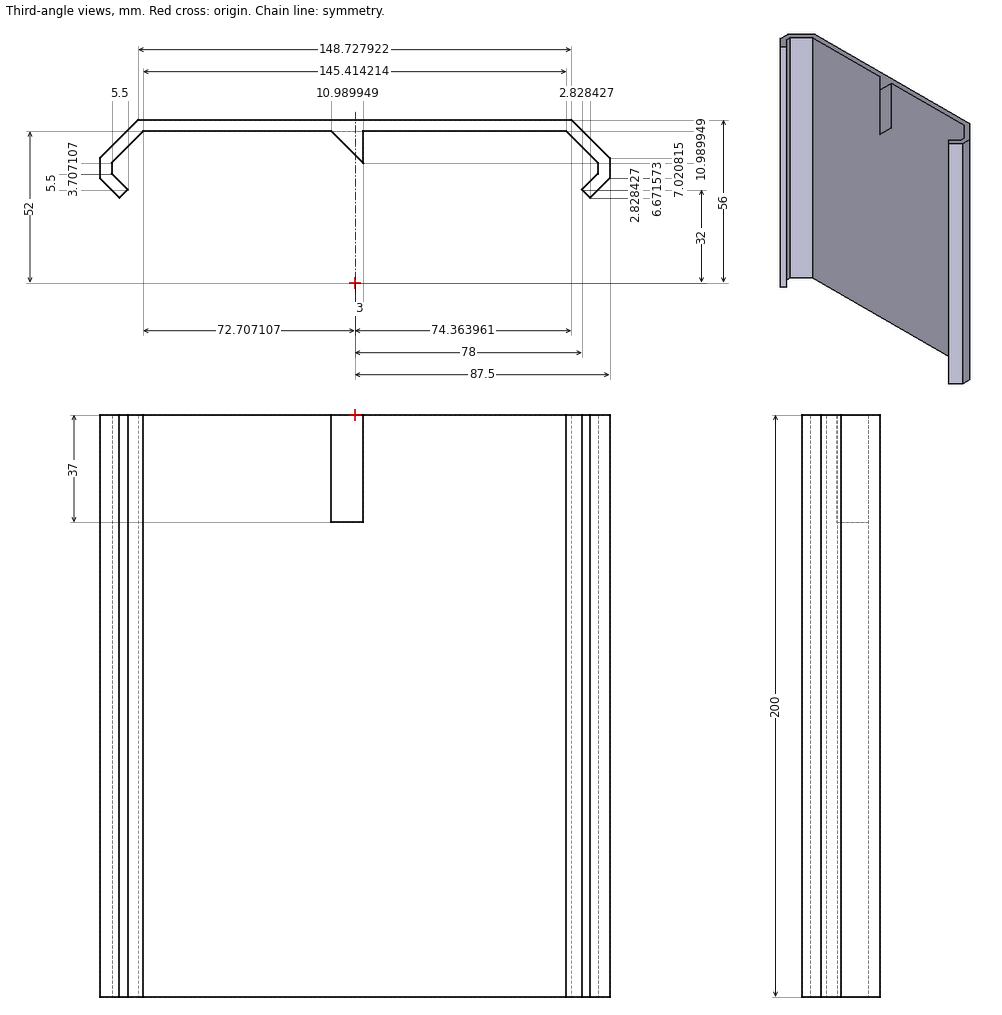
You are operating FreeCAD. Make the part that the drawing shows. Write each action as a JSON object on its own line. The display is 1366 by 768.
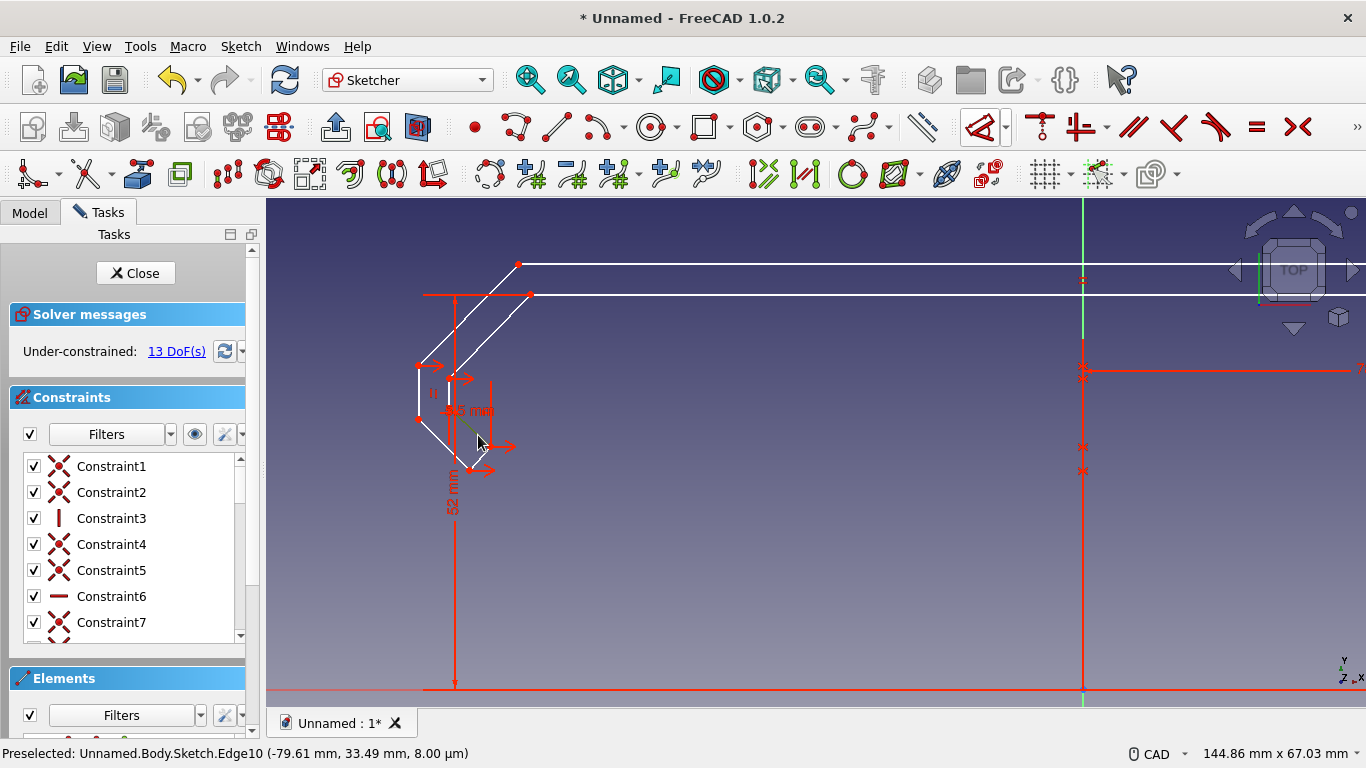
{"action": "key", "text": "i"}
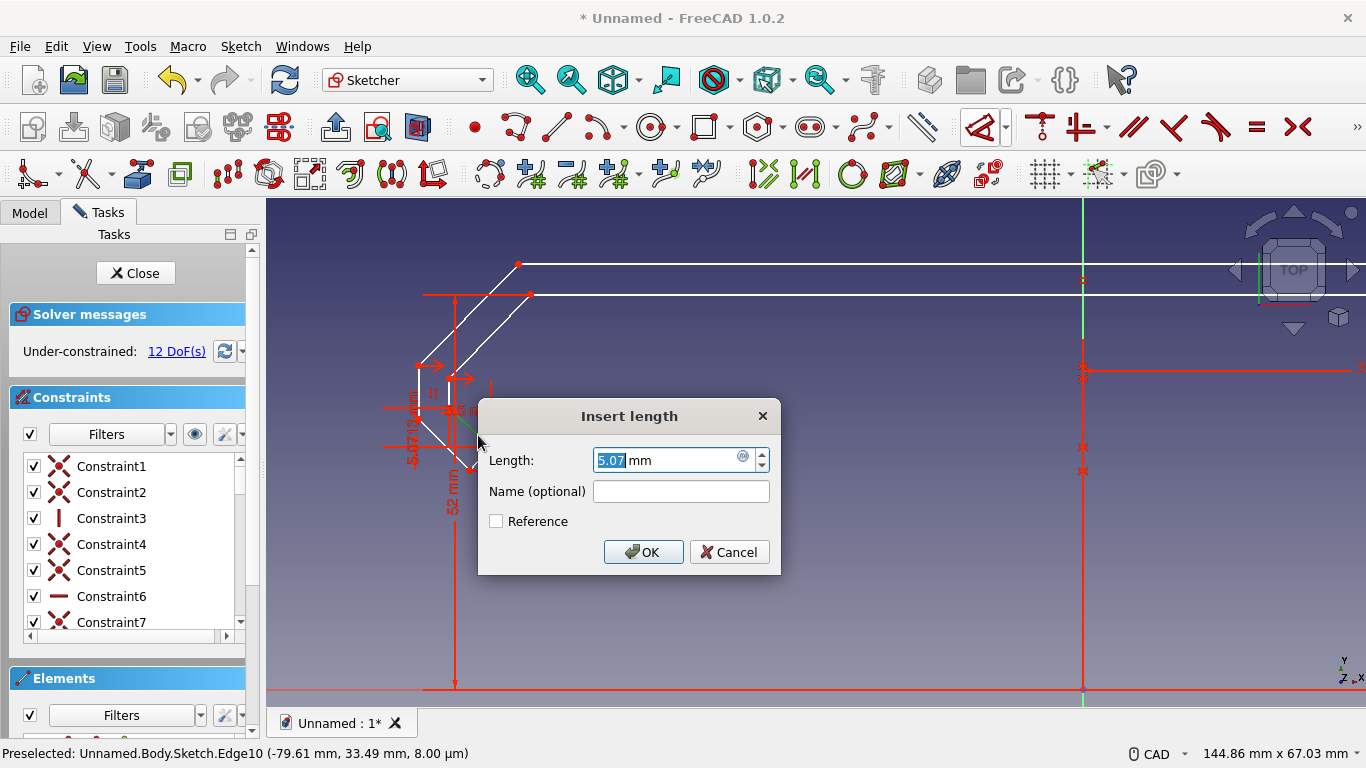
{"action": "type", "text": "5.5"}
{"action": "key", "text": "Return"}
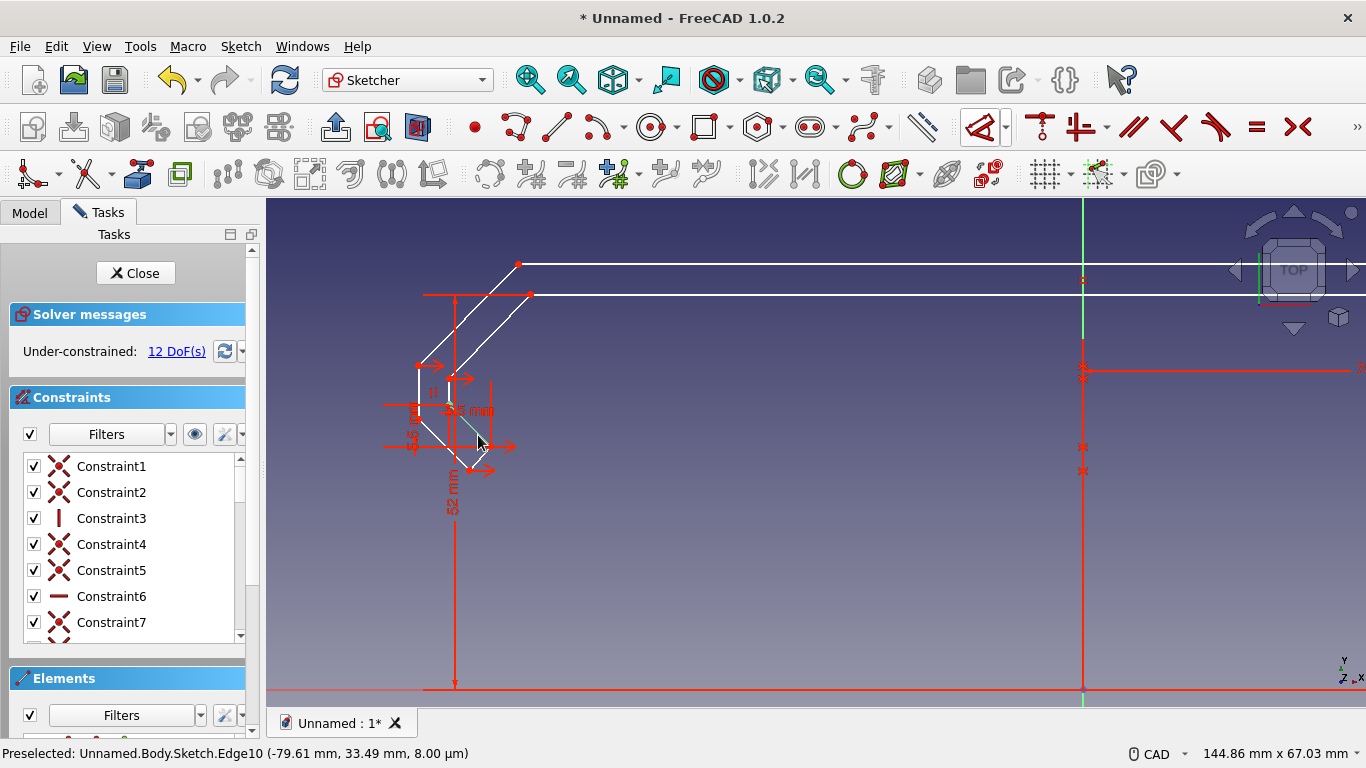
{"action": "scroll", "coordinate": [474, 432], "scroll_direction": "down", "scroll_amount": 4}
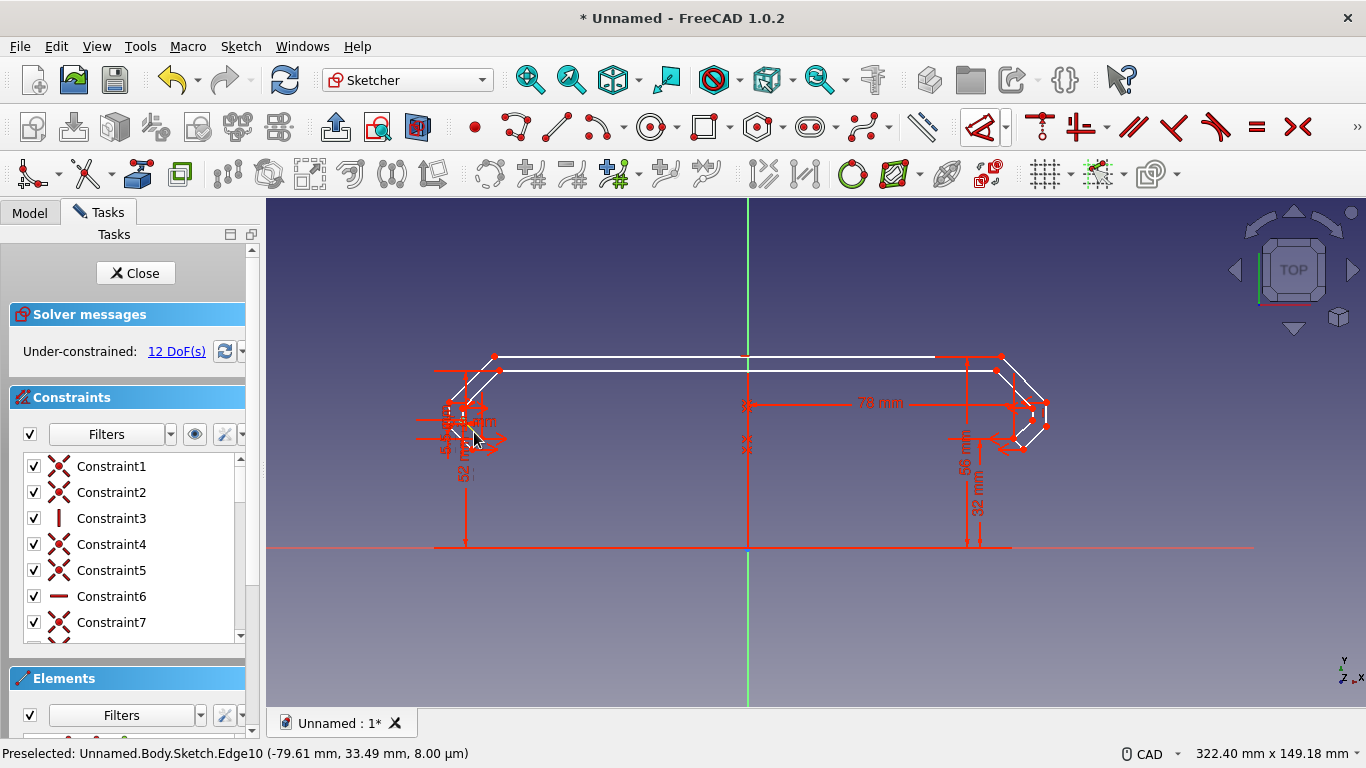
{"action": "scroll", "coordinate": [1027, 426], "scroll_direction": "up", "scroll_amount": 4}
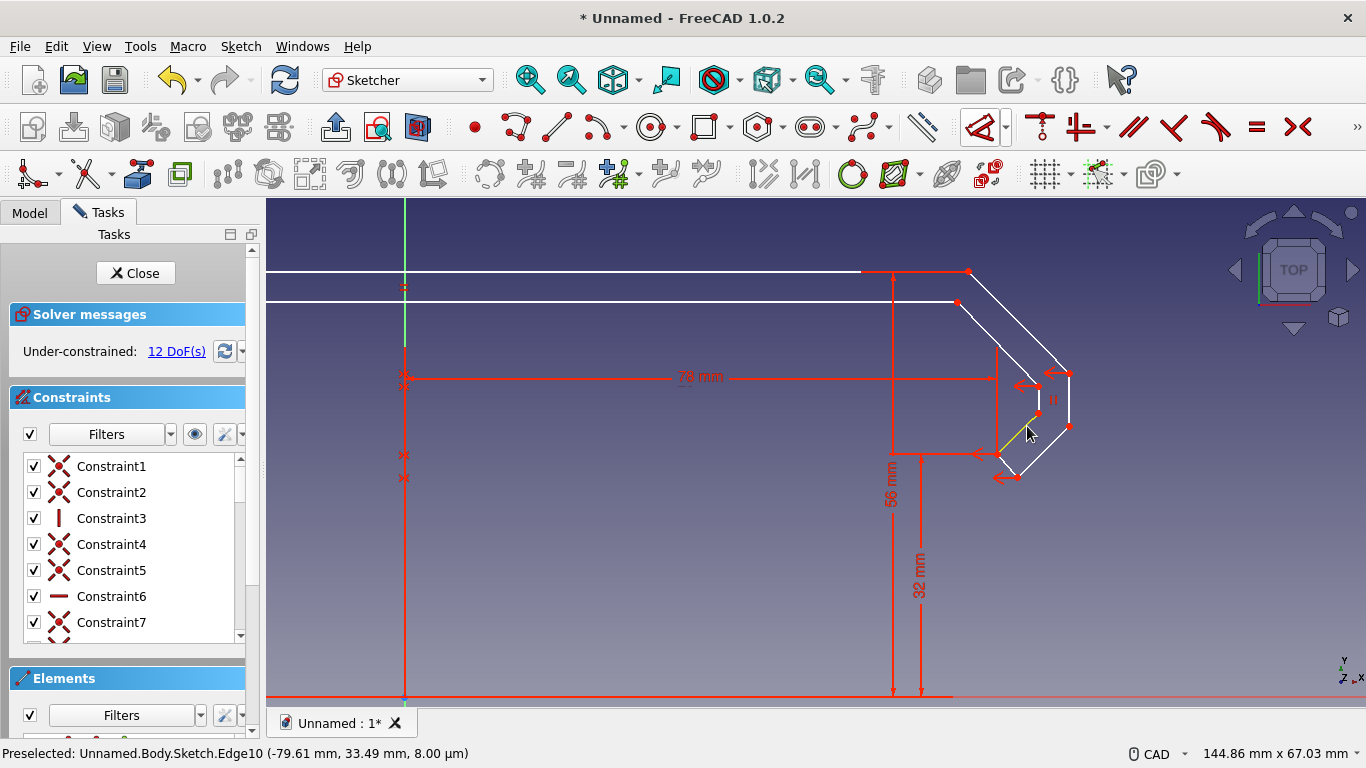
{"action": "left_click", "coordinate": [1026, 426]}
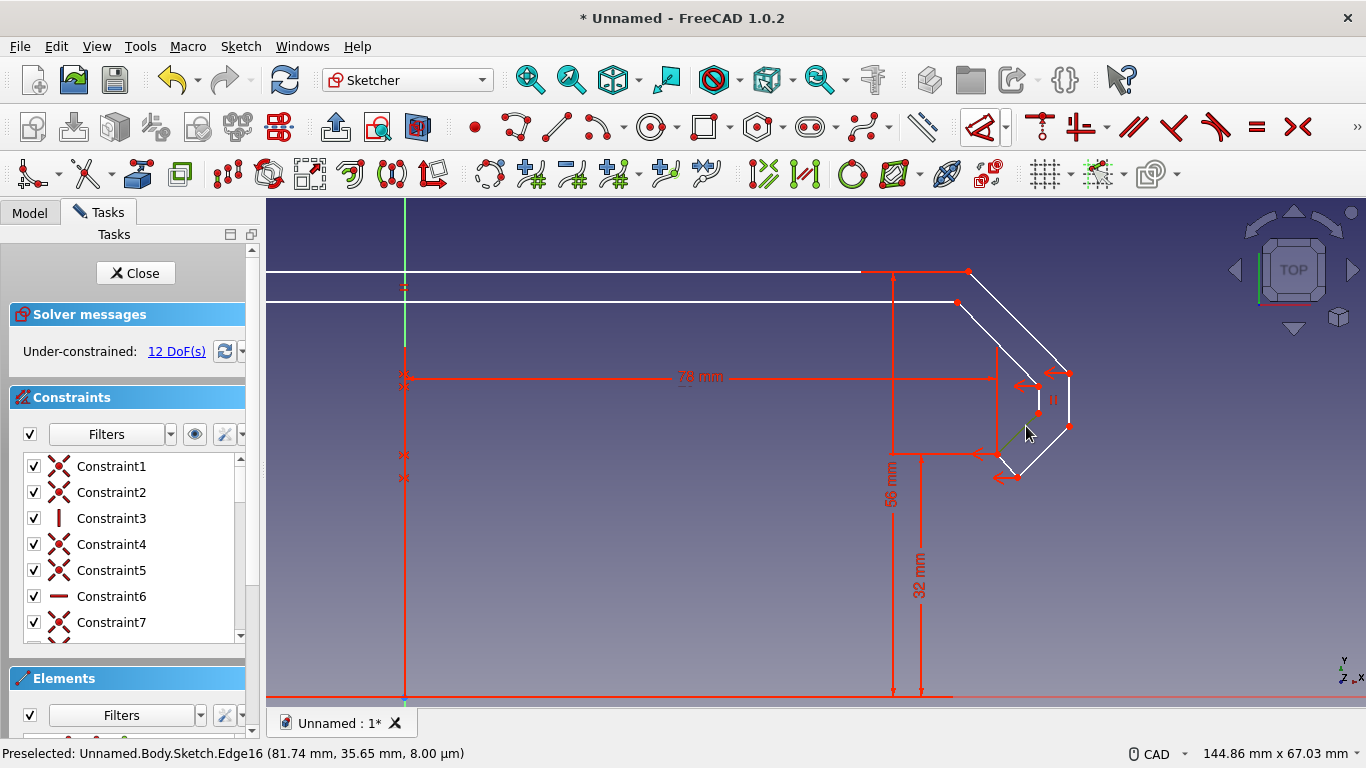
{"action": "key", "text": "i"}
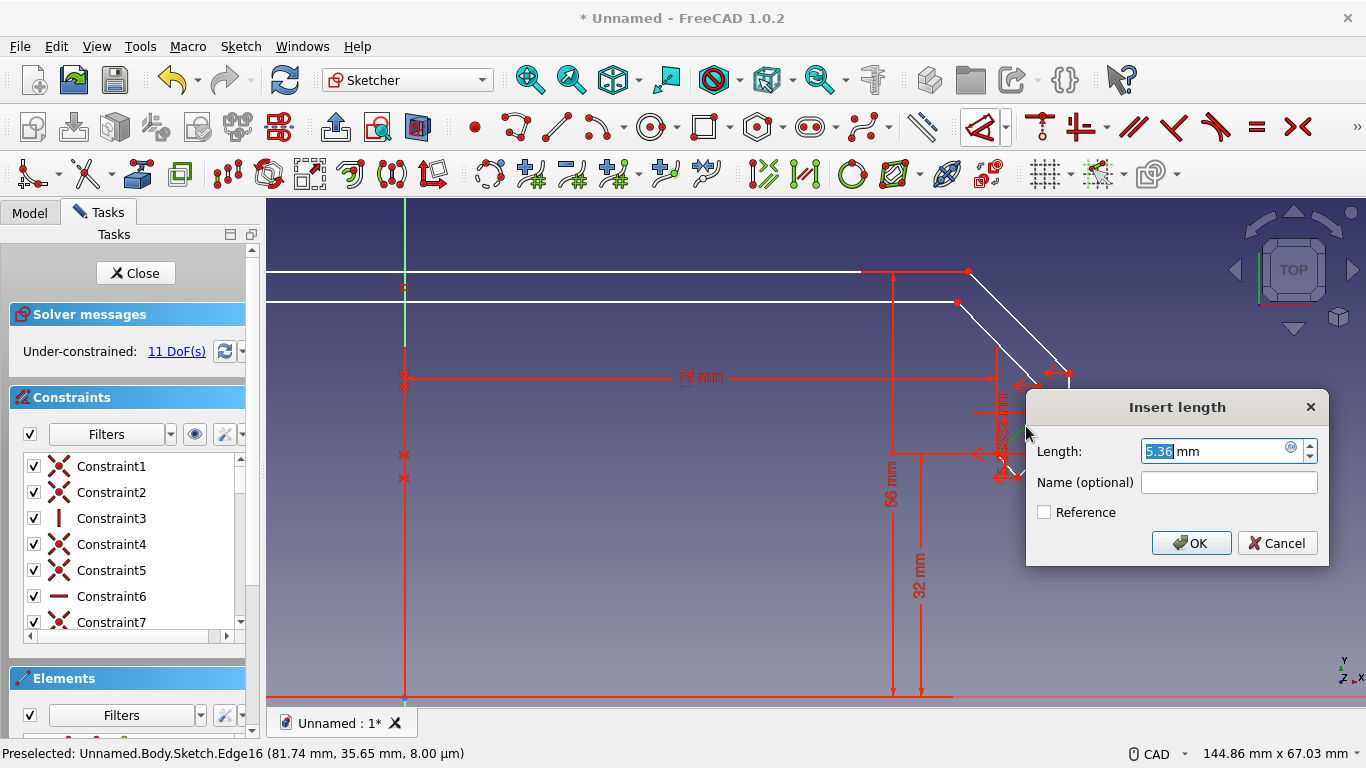
{"action": "type", "text": "5.5"}
{"action": "key", "text": "Return"}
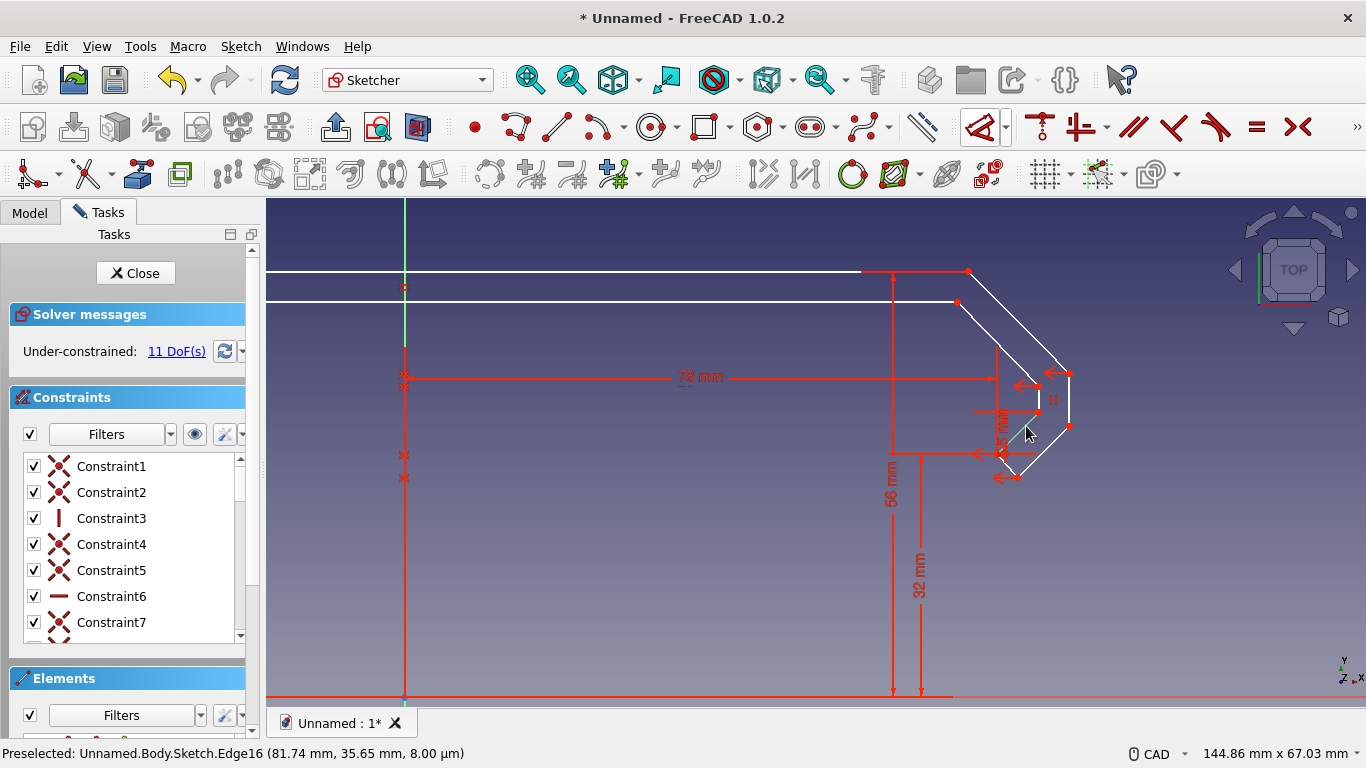
{"action": "left_click", "coordinate": [1069, 427]}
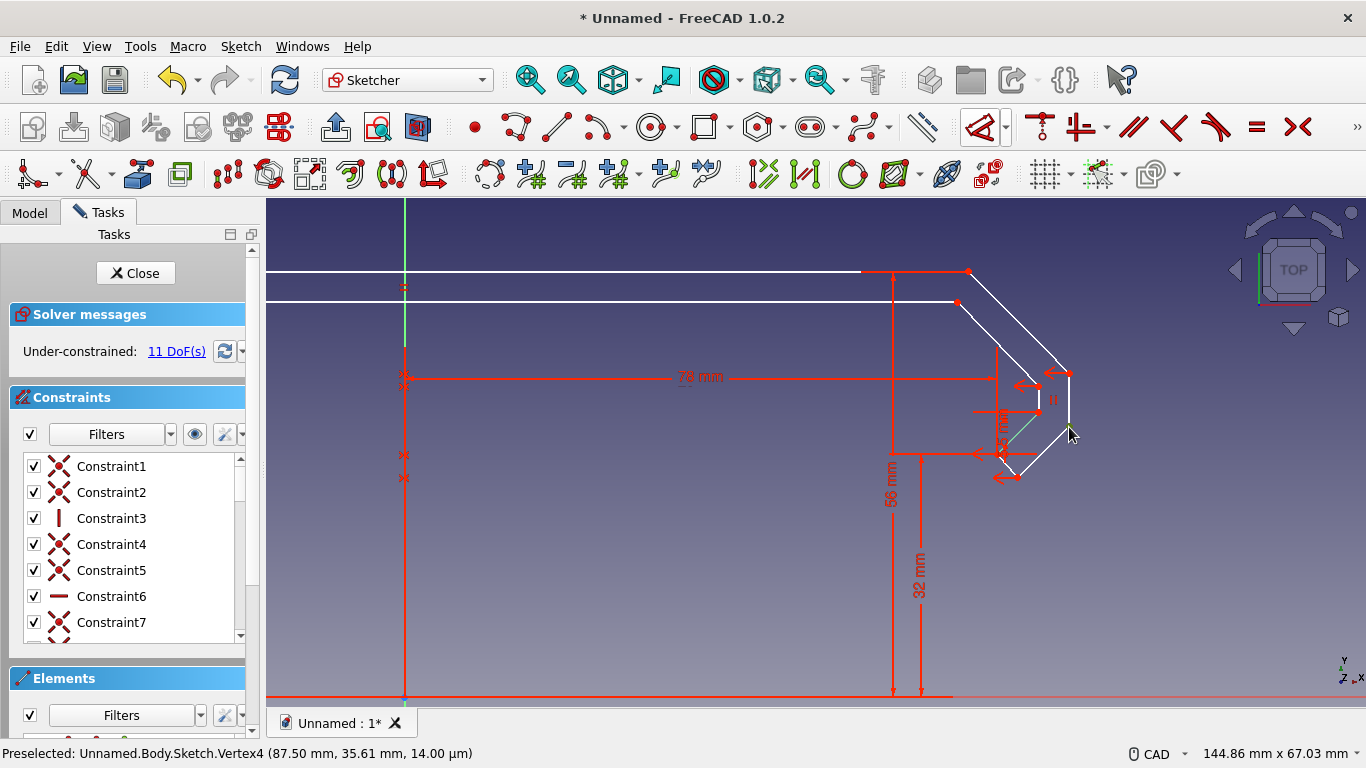
{"action": "key", "text": "l"}